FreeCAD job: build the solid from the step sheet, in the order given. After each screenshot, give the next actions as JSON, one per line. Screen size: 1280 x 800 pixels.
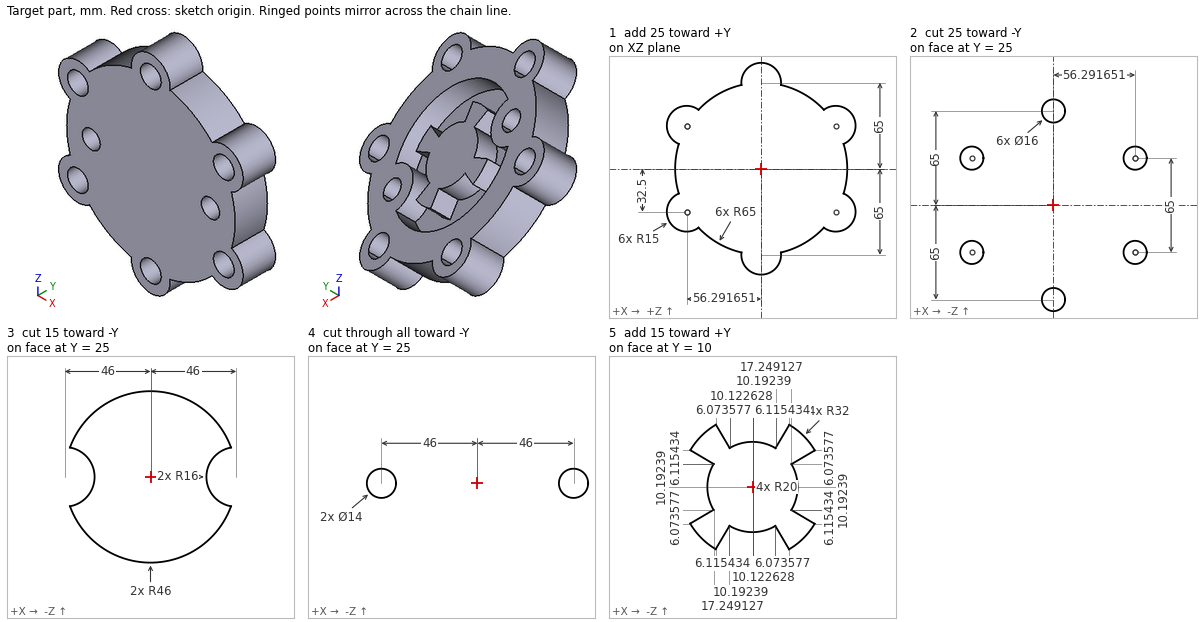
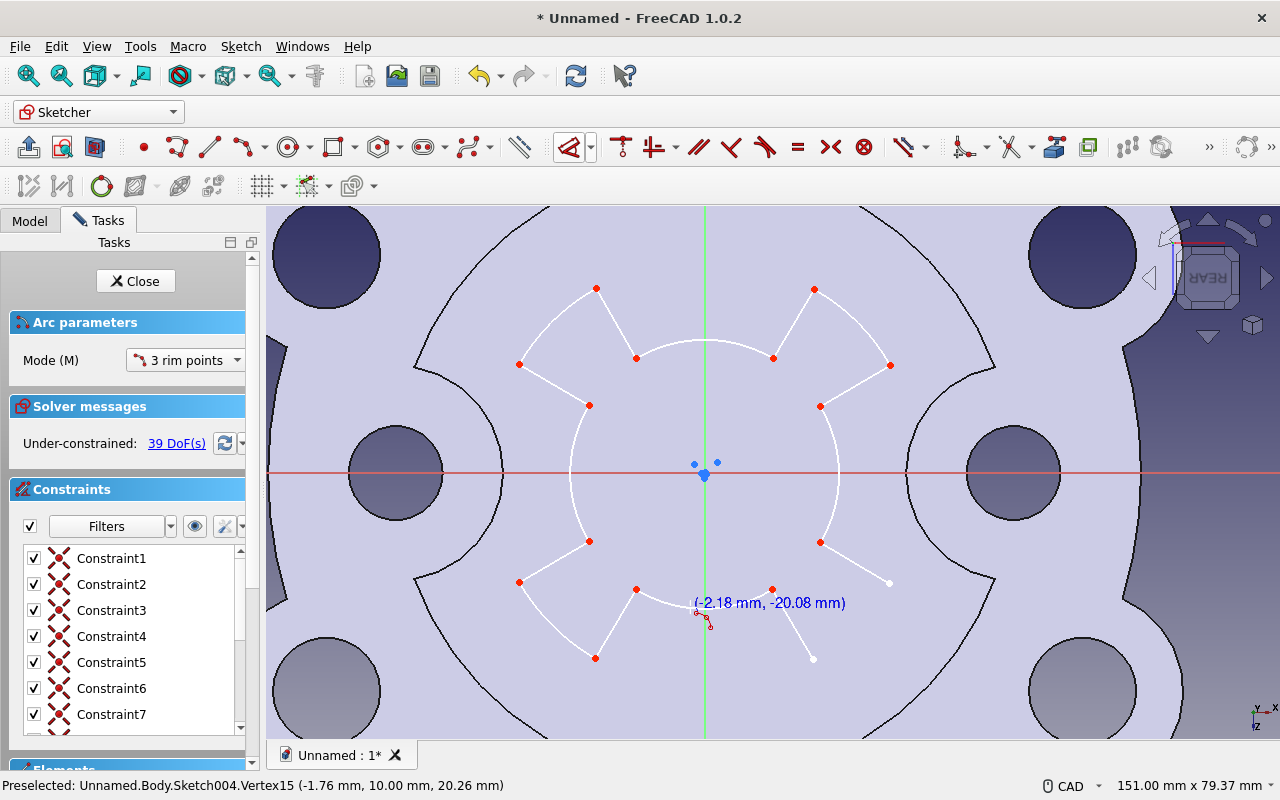
{"action": "left_click", "coordinate": [813, 660]}
{"action": "left_click", "coordinate": [889, 584]}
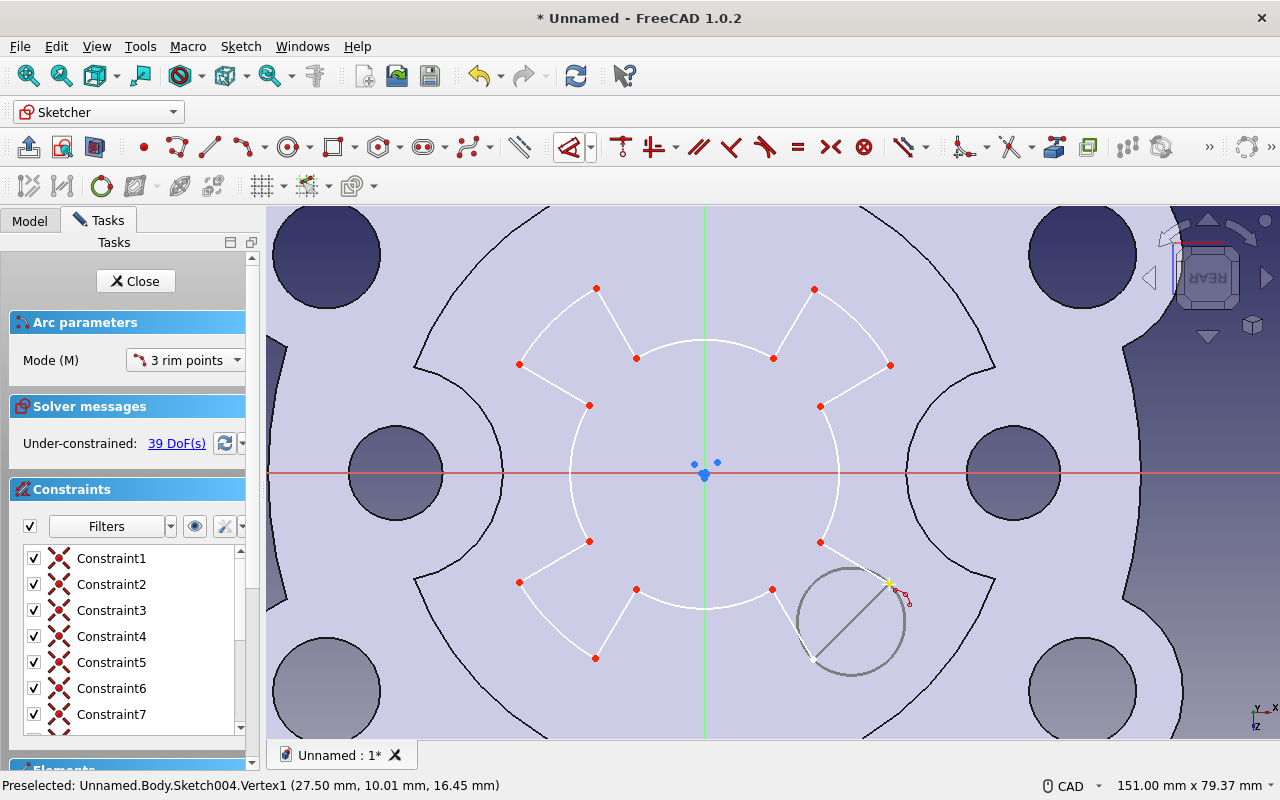
{"action": "scroll", "coordinate": [856, 625], "scroll_direction": "up", "scroll_amount": 5}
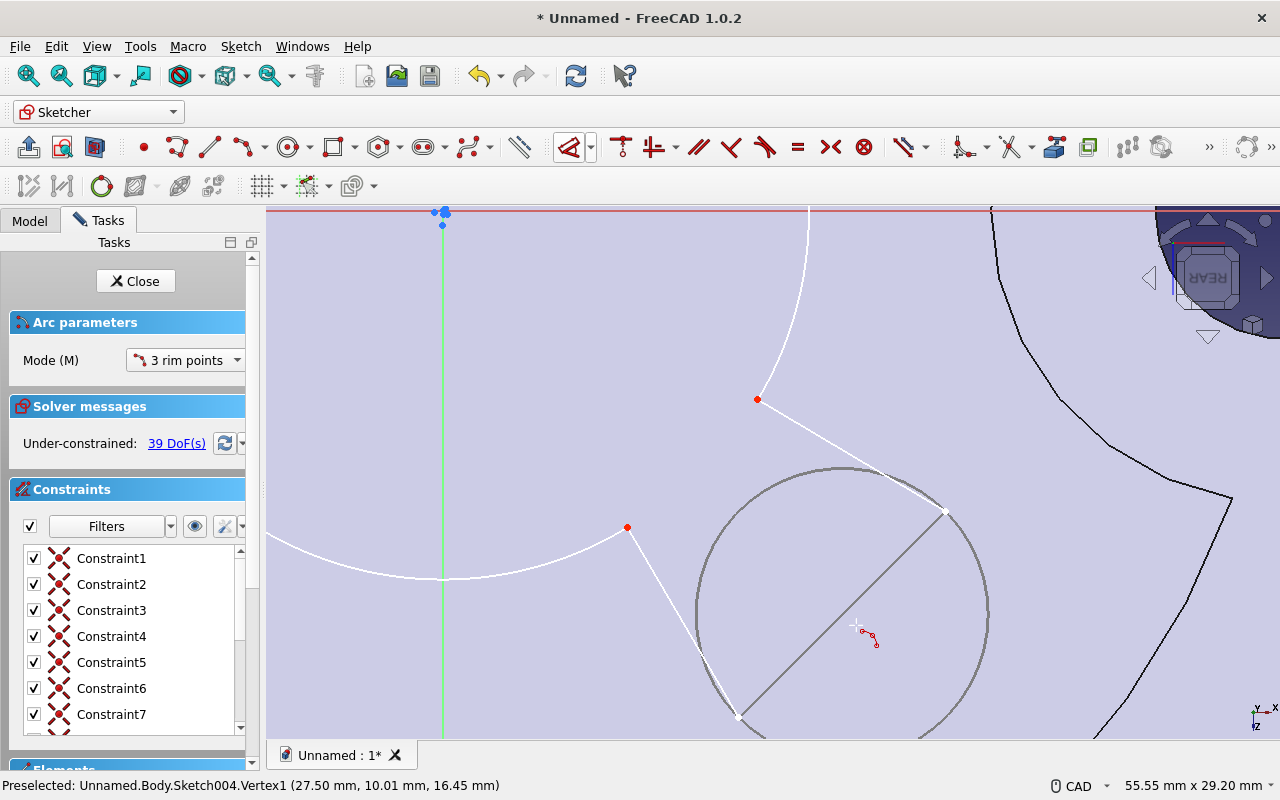
{"action": "left_click", "coordinate": [856, 625]}
{"action": "key", "text": "Escape"}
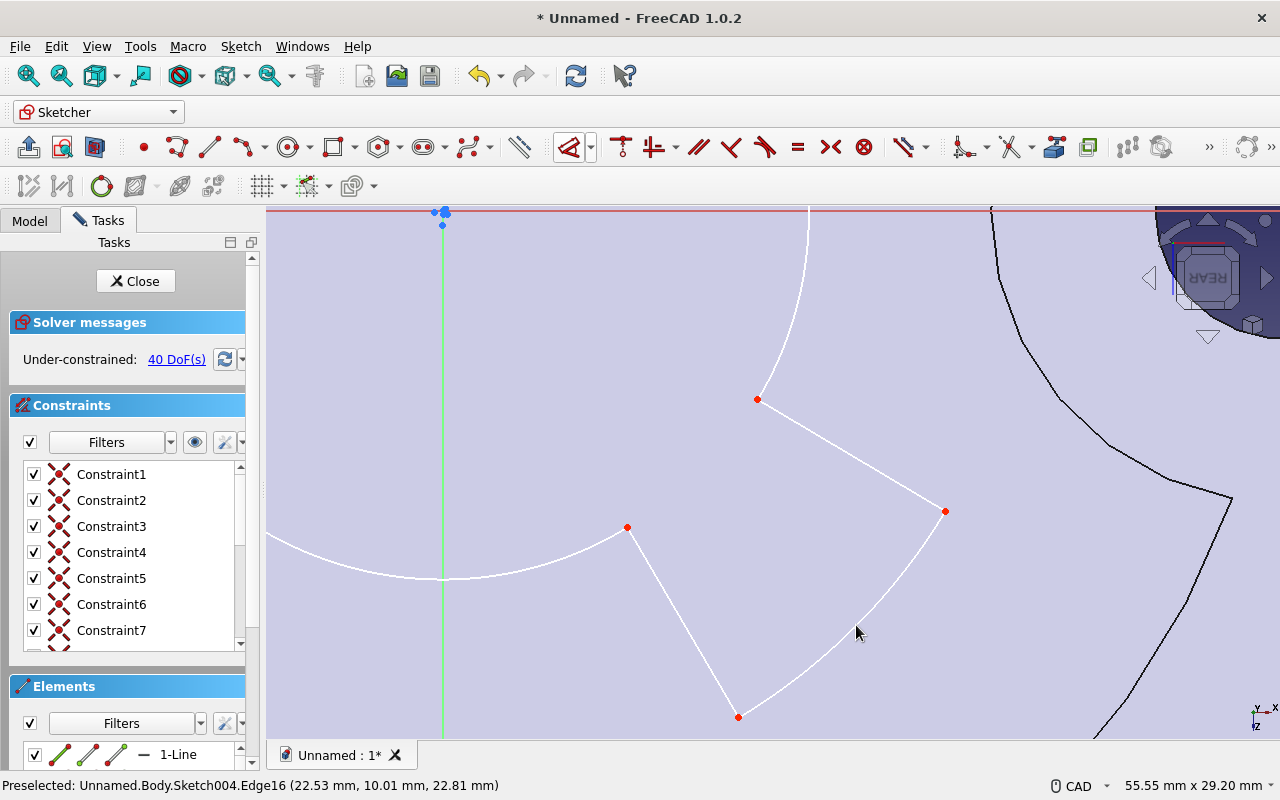
{"action": "left_click", "coordinate": [800, 292]}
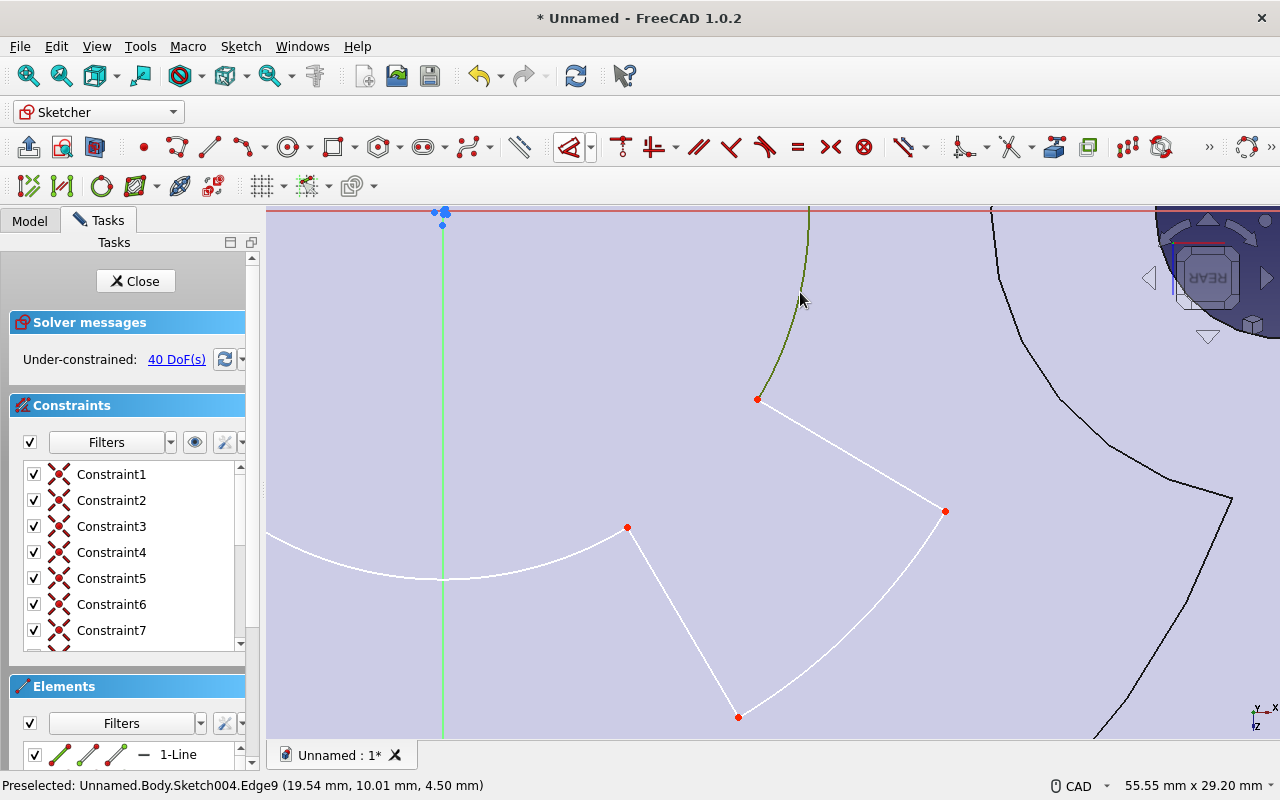
{"action": "scroll", "coordinate": [856, 625], "scroll_direction": "down", "scroll_amount": 5}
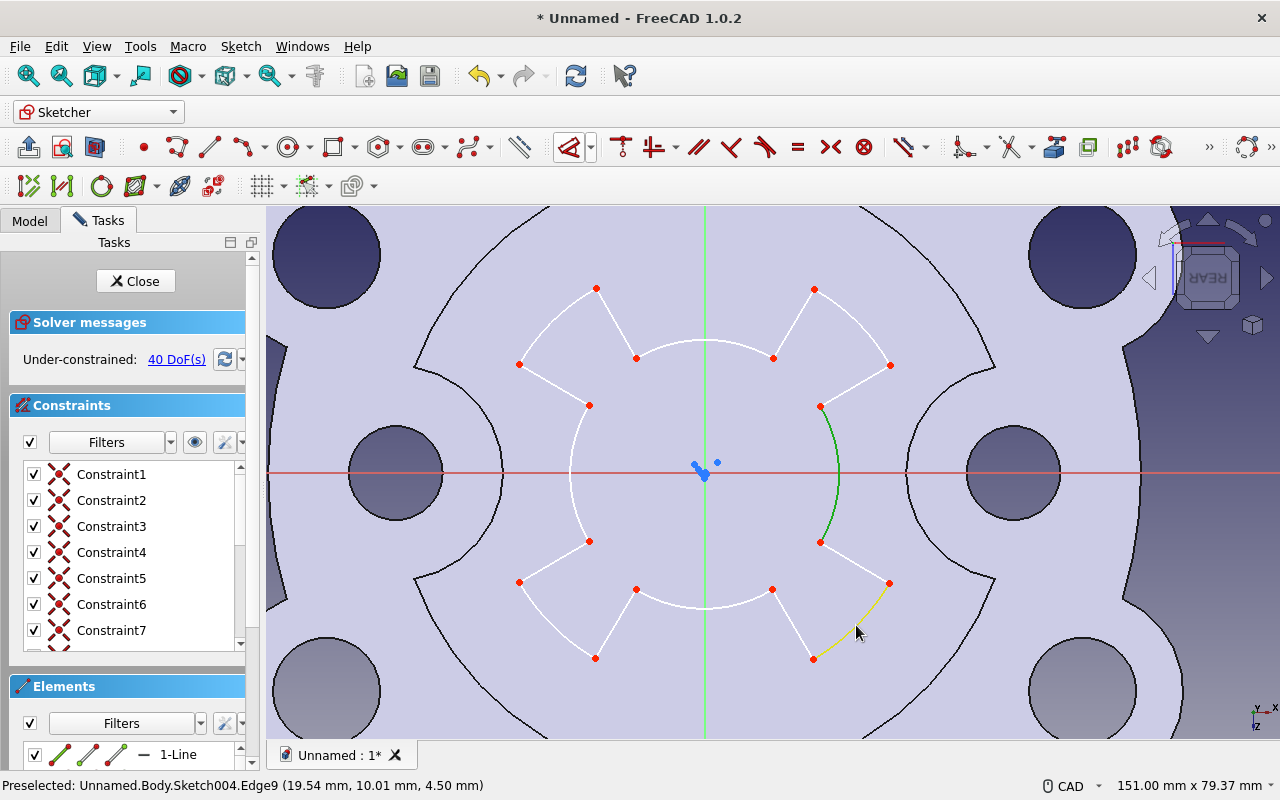
{"action": "left_click", "coordinate": [872, 339]}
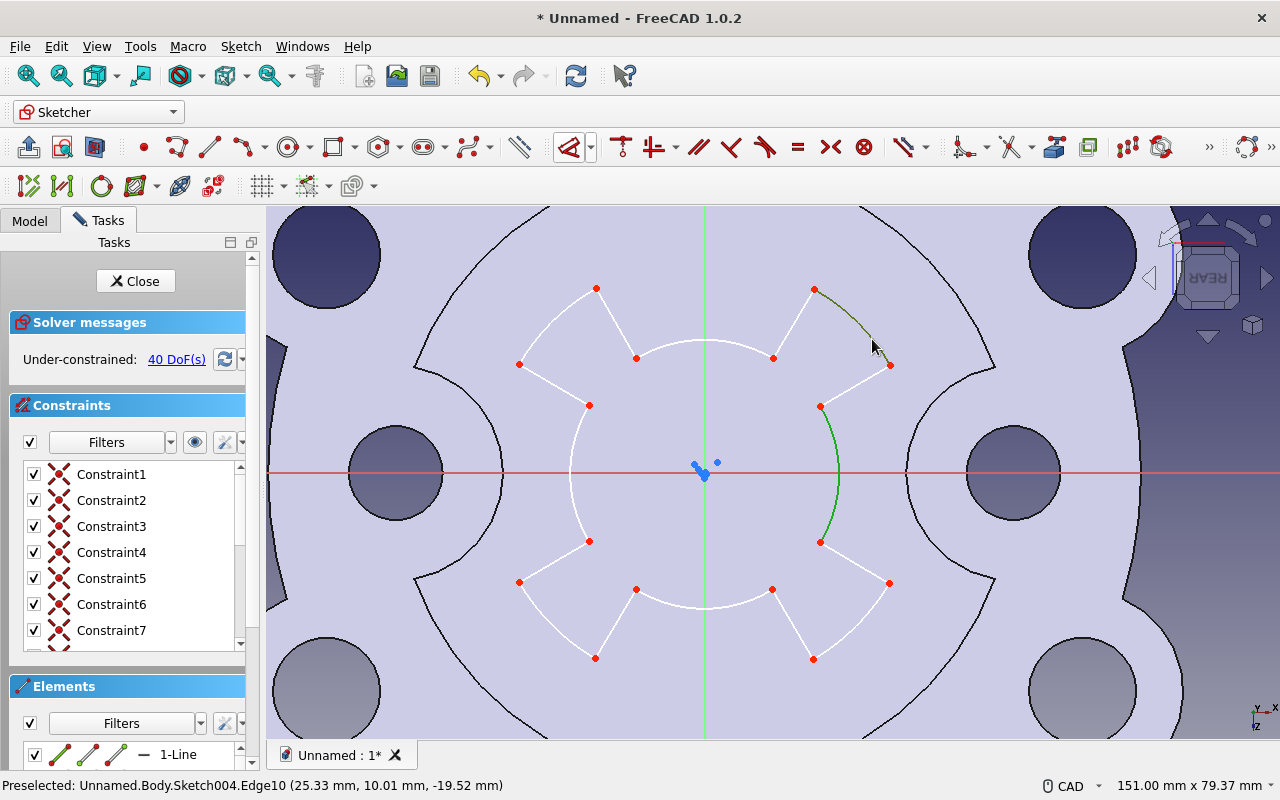
{"action": "left_click", "coordinate": [621, 148]}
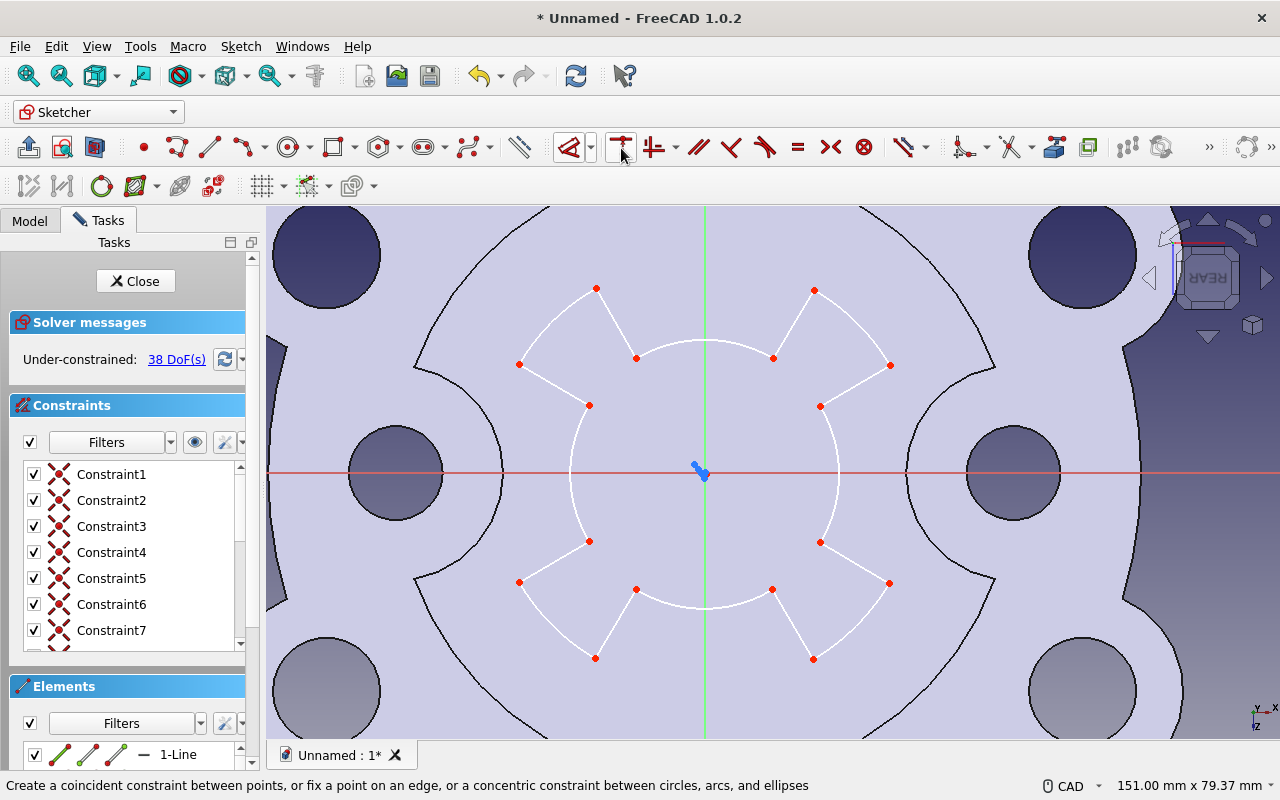
{"action": "left_click", "coordinate": [836, 503]}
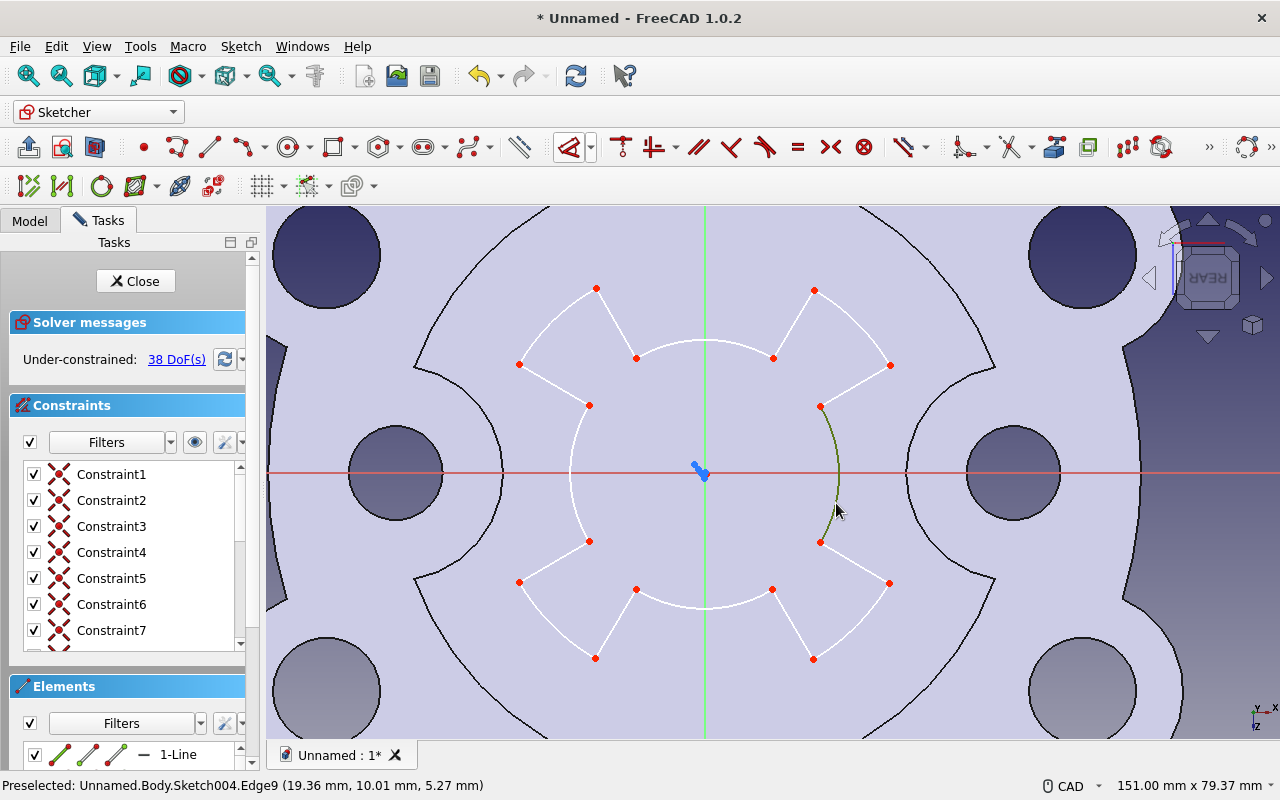
{"action": "left_click", "coordinate": [733, 343]}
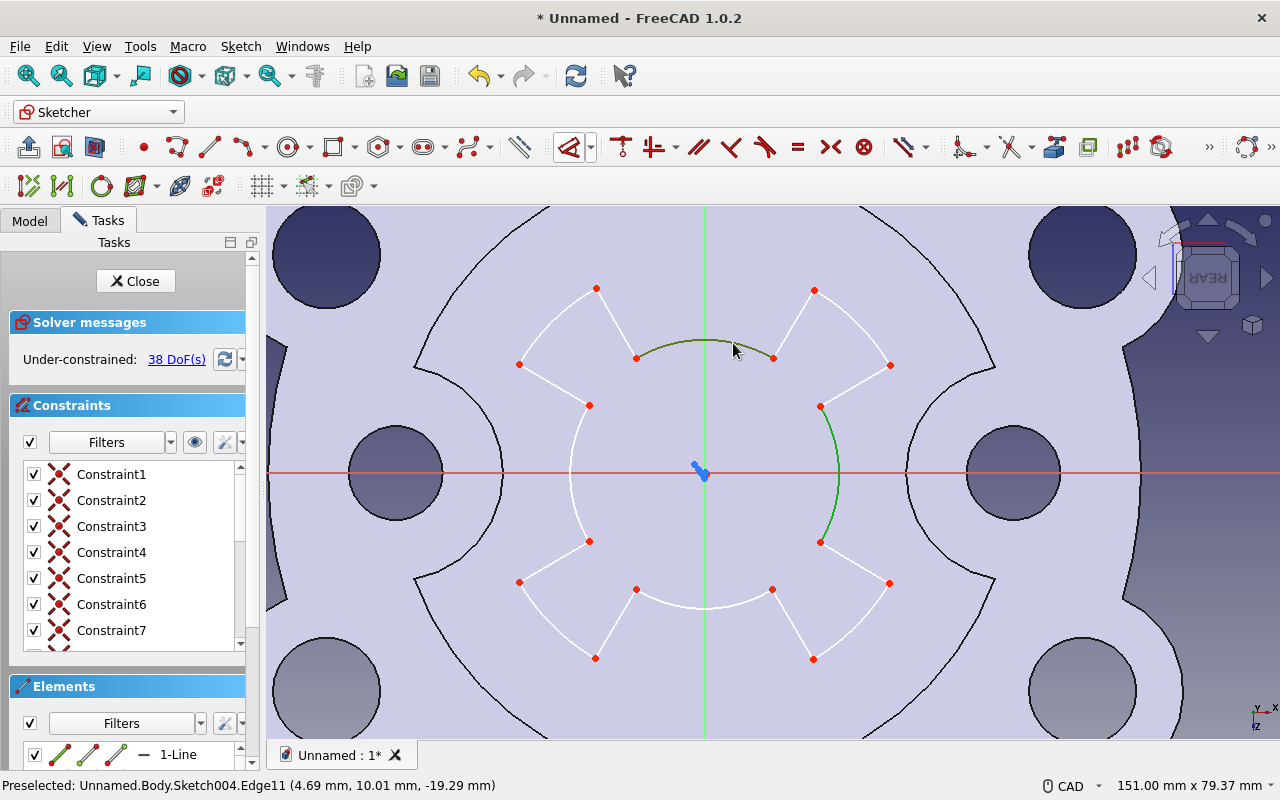
{"action": "left_click", "coordinate": [621, 148]}